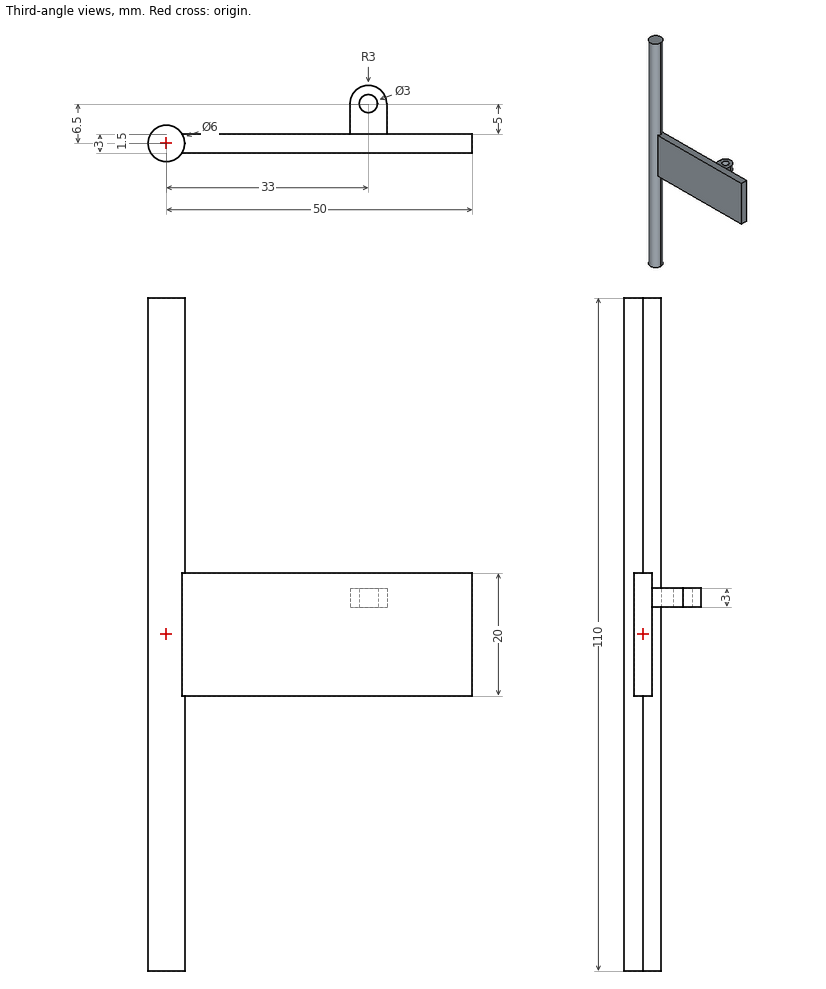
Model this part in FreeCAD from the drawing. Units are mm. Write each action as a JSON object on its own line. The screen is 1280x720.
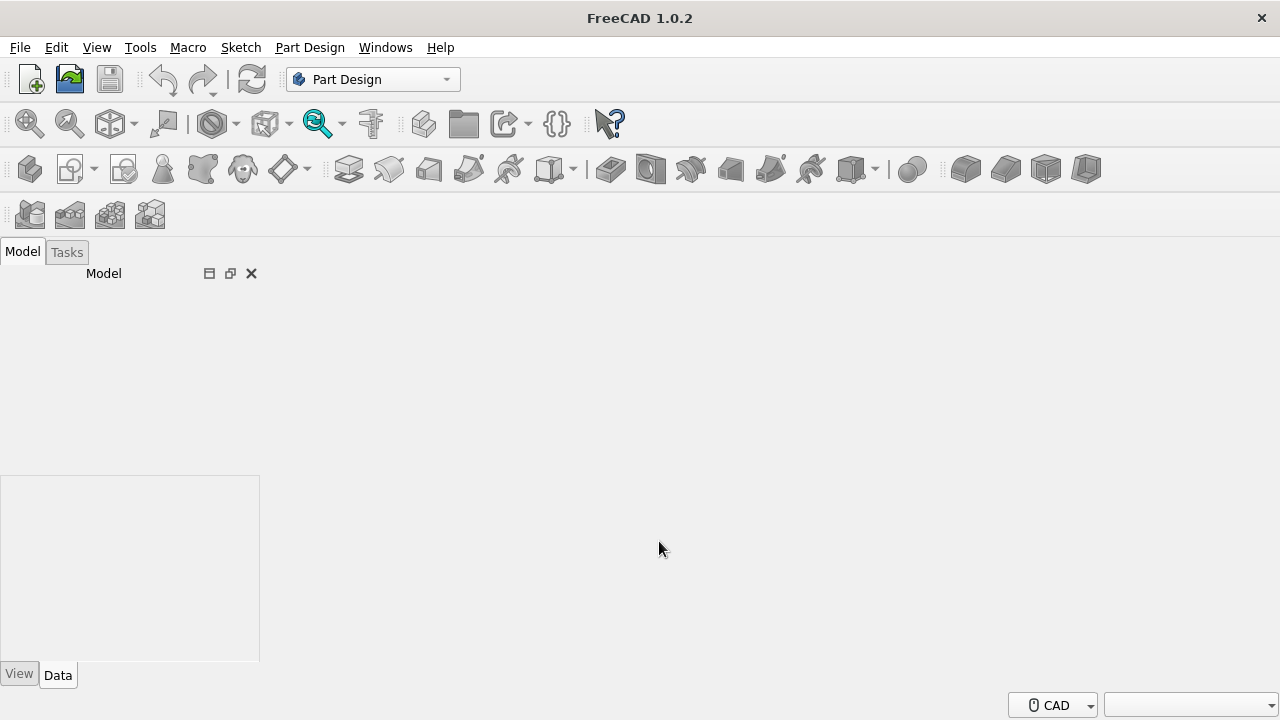
{"action": "left_click", "coordinate": [30, 80]}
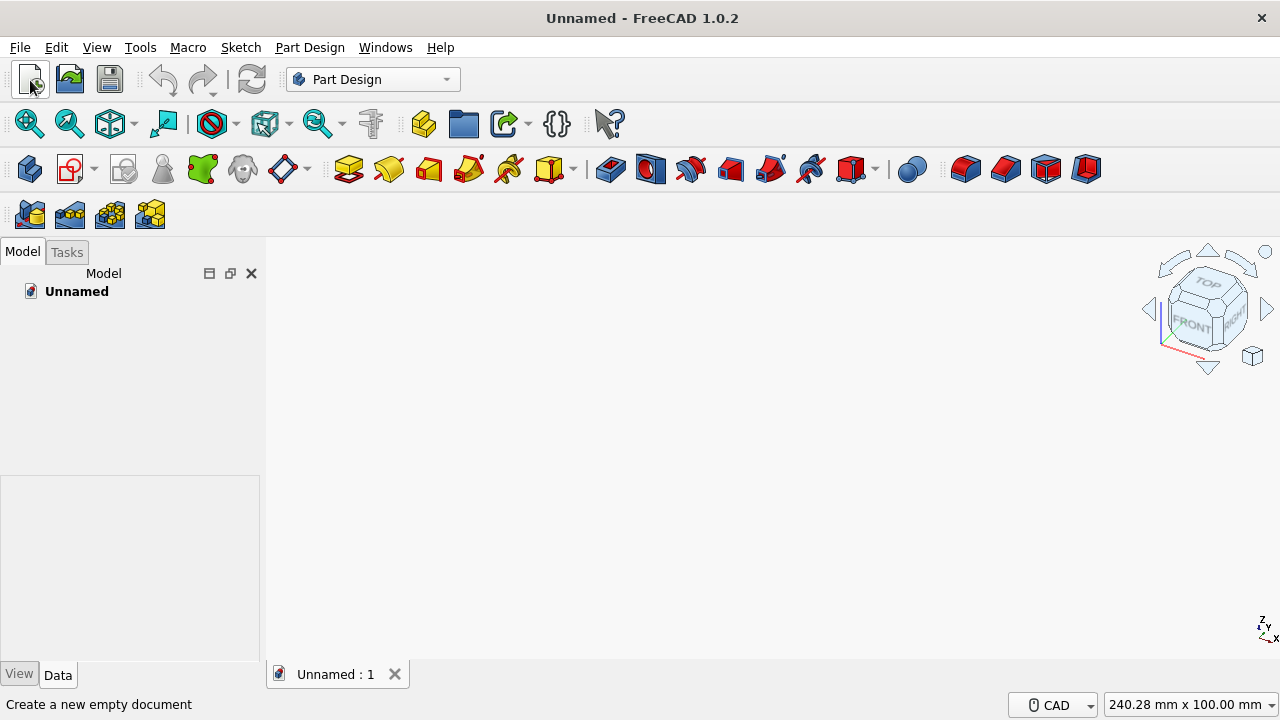
{"action": "left_click", "coordinate": [70, 170]}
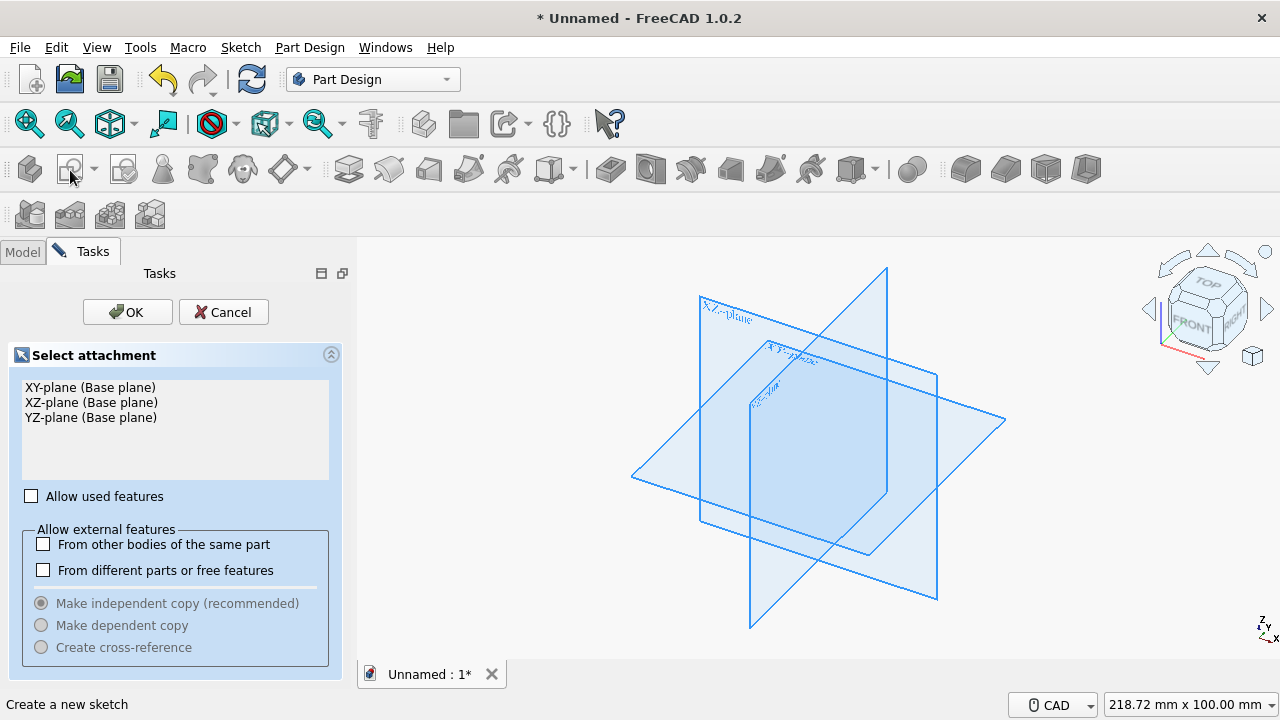
{"action": "left_click", "coordinate": [82, 388]}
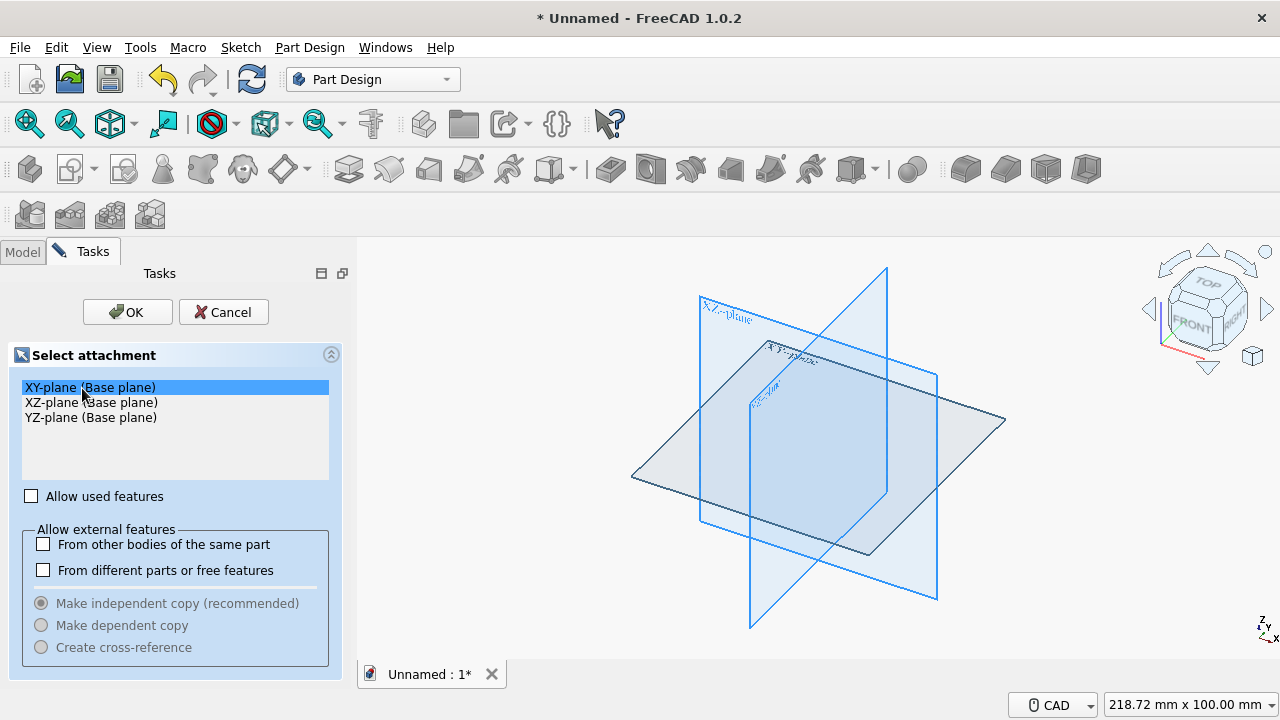
{"action": "left_click", "coordinate": [128, 312]}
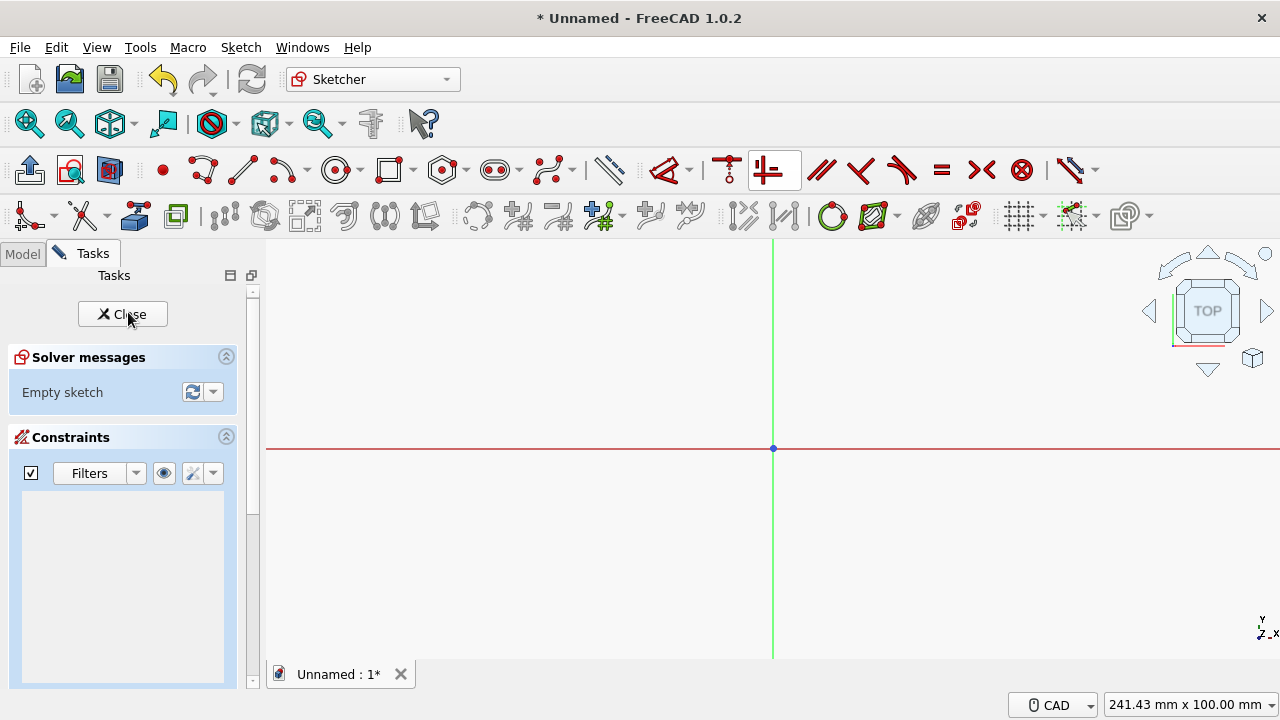
{"action": "scroll", "coordinate": [780, 449], "scroll_direction": "up", "scroll_amount": 12}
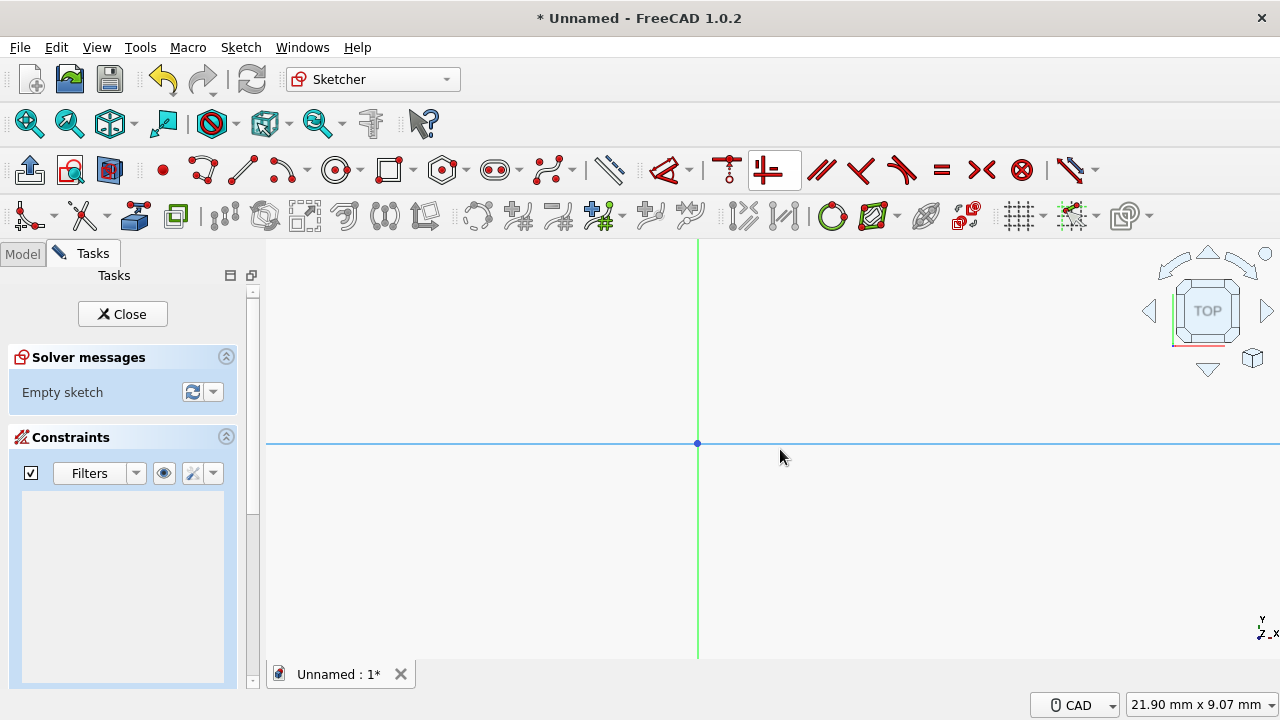
{"action": "left_click", "coordinate": [336, 170]}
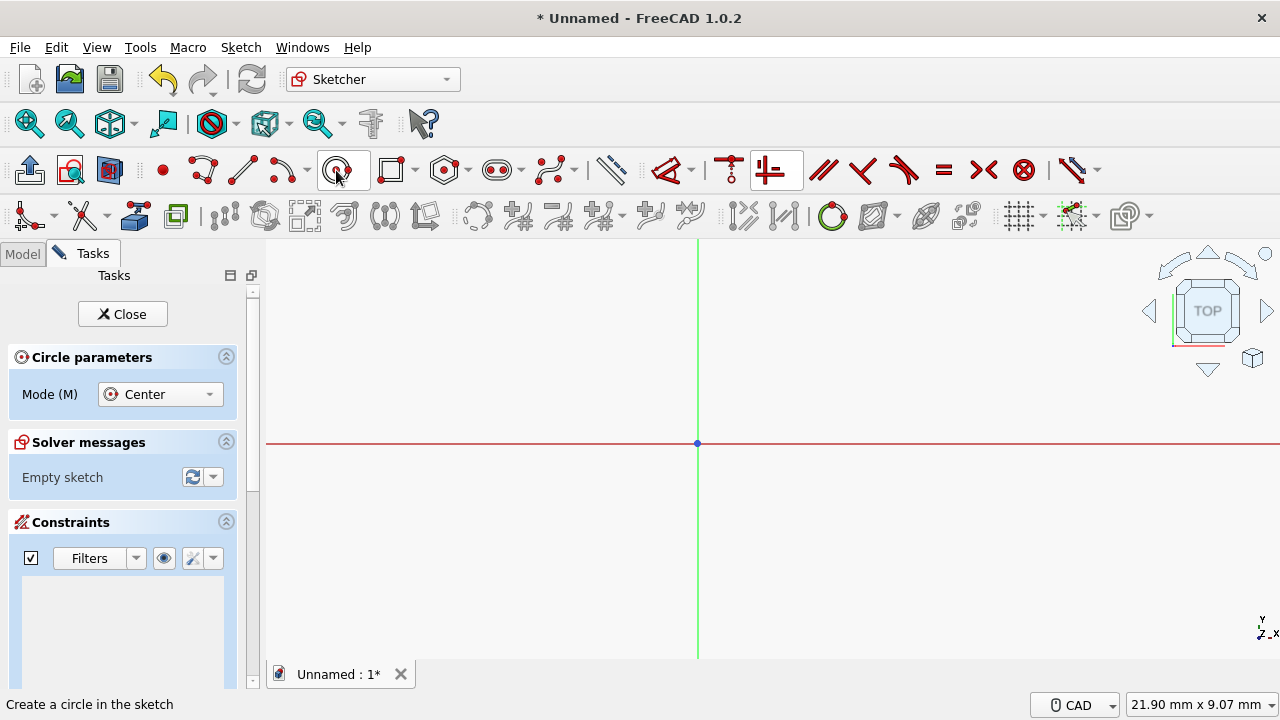
{"action": "left_click", "coordinate": [698, 444]}
{"action": "left_click", "coordinate": [796, 346]}
{"action": "key", "text": "Escape"}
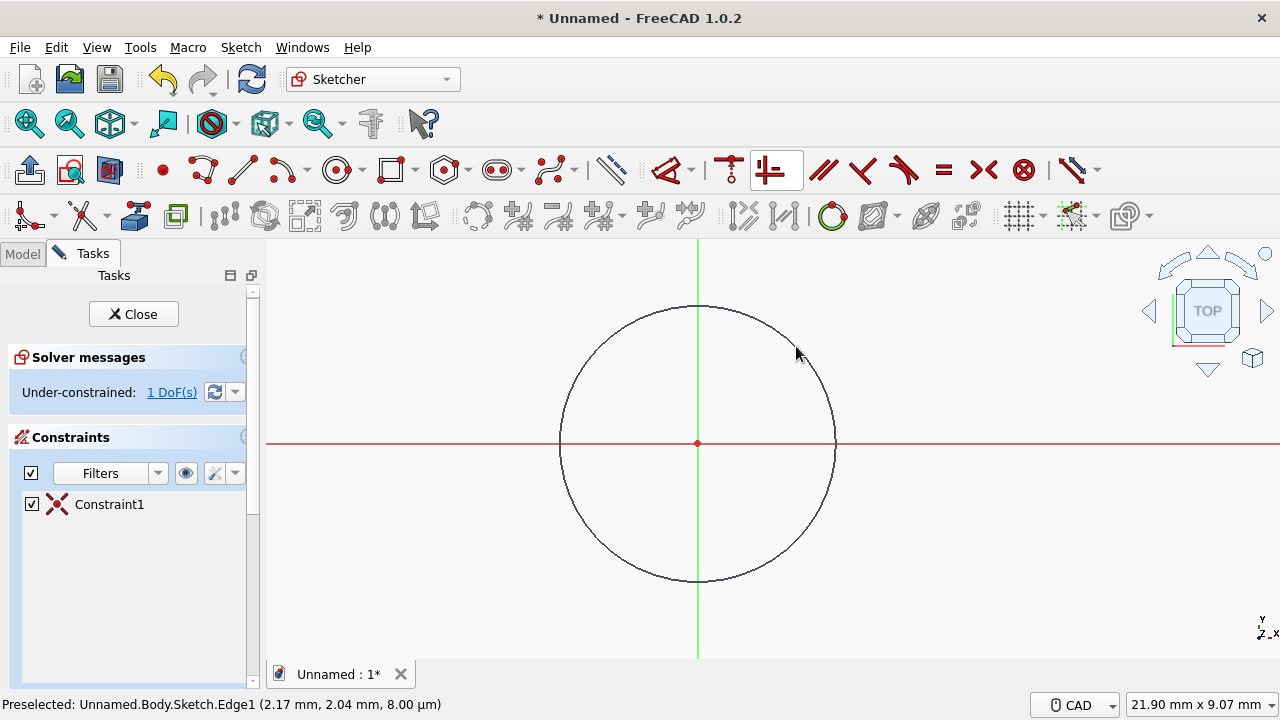
{"action": "left_click", "coordinate": [795, 346]}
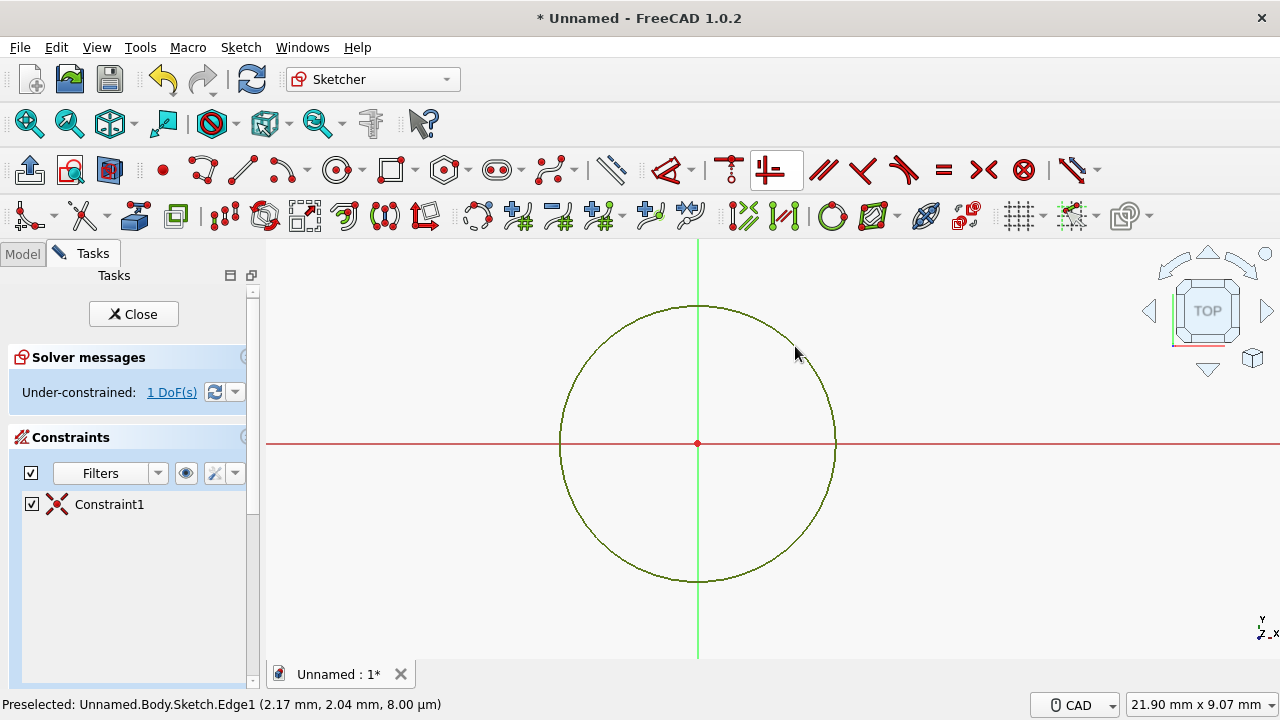
{"action": "left_click", "coordinate": [694, 170]}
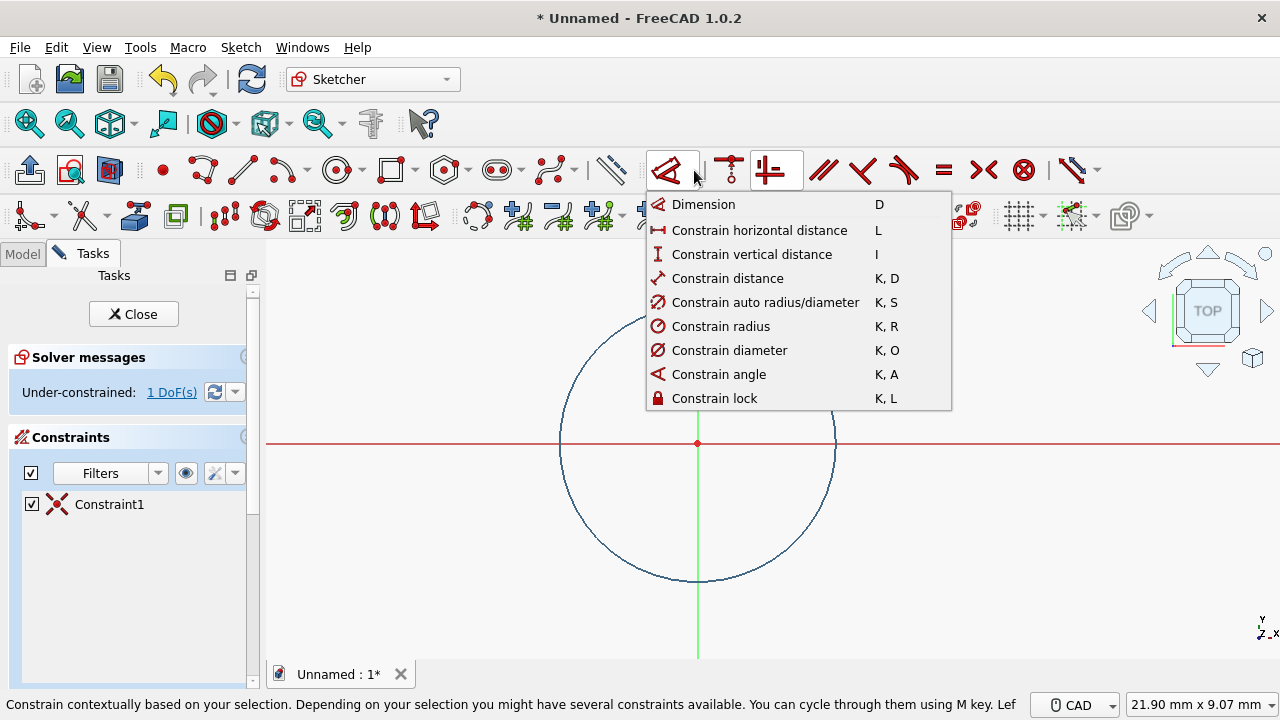
{"action": "left_click", "coordinate": [799, 350]}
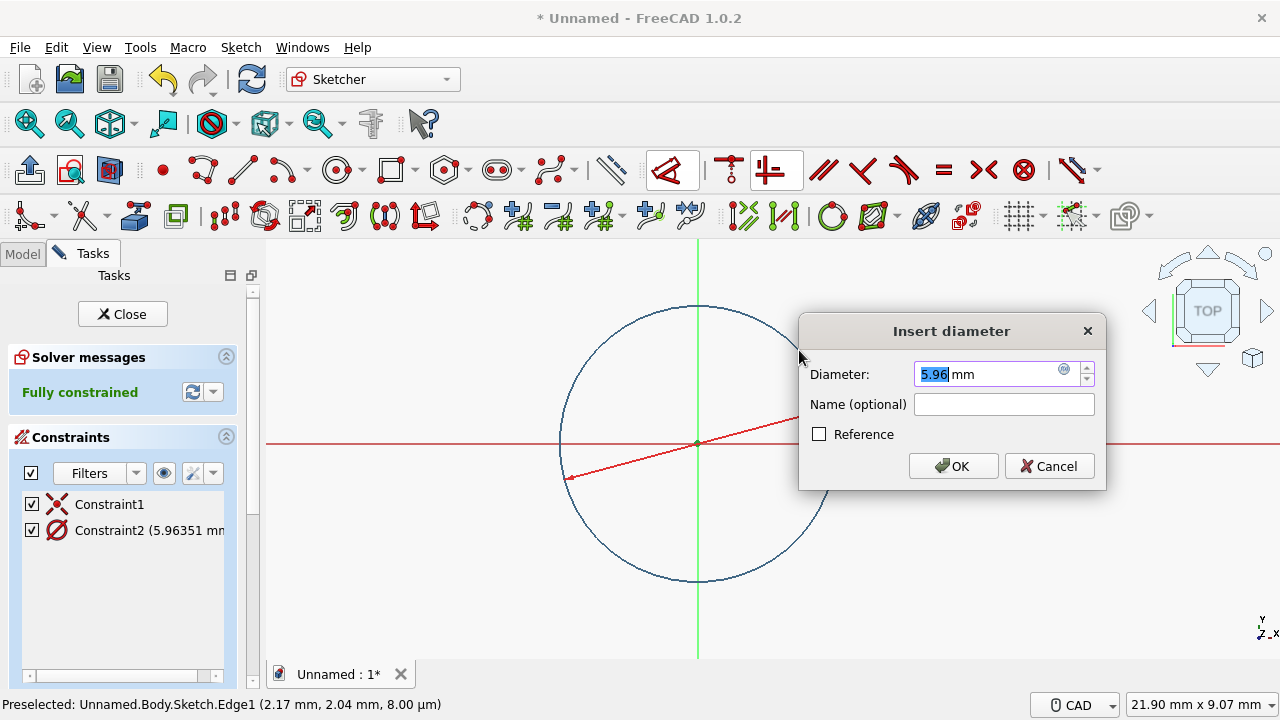
{"action": "type", "text": "6"}
{"action": "key", "text": "Return"}